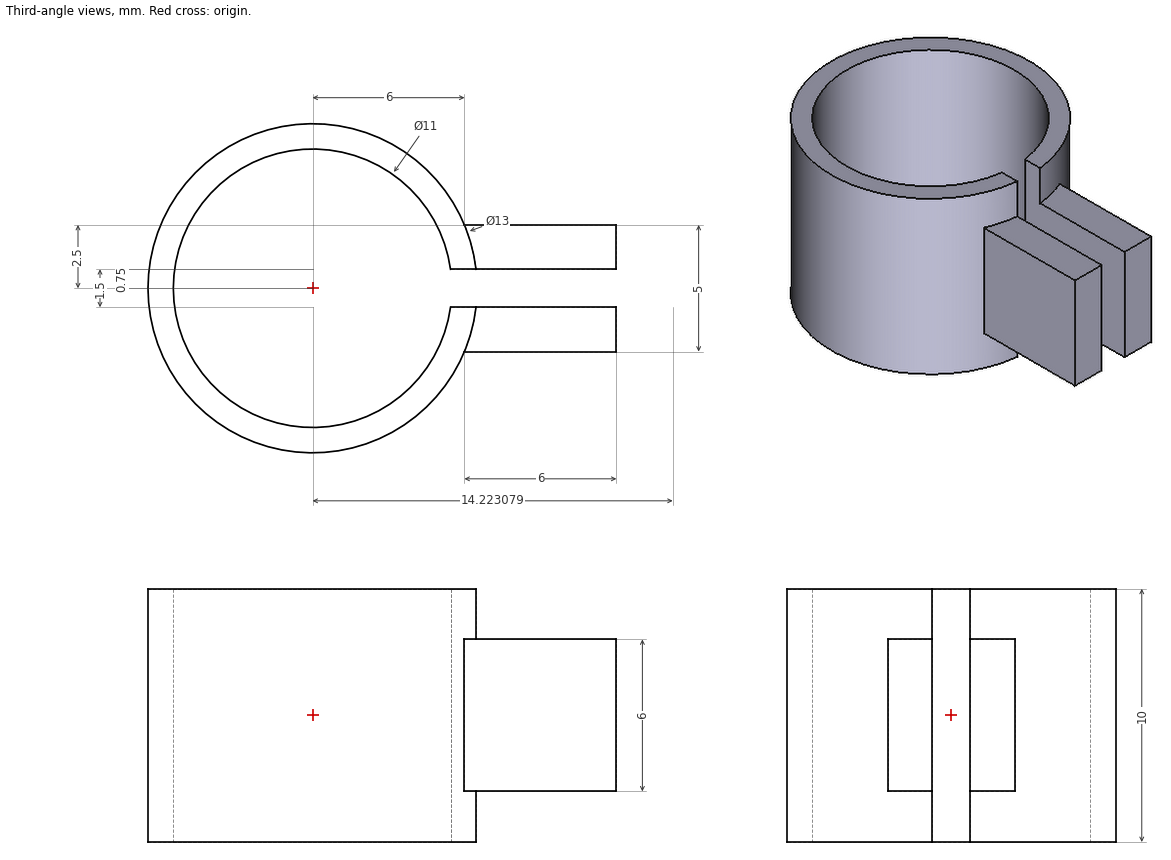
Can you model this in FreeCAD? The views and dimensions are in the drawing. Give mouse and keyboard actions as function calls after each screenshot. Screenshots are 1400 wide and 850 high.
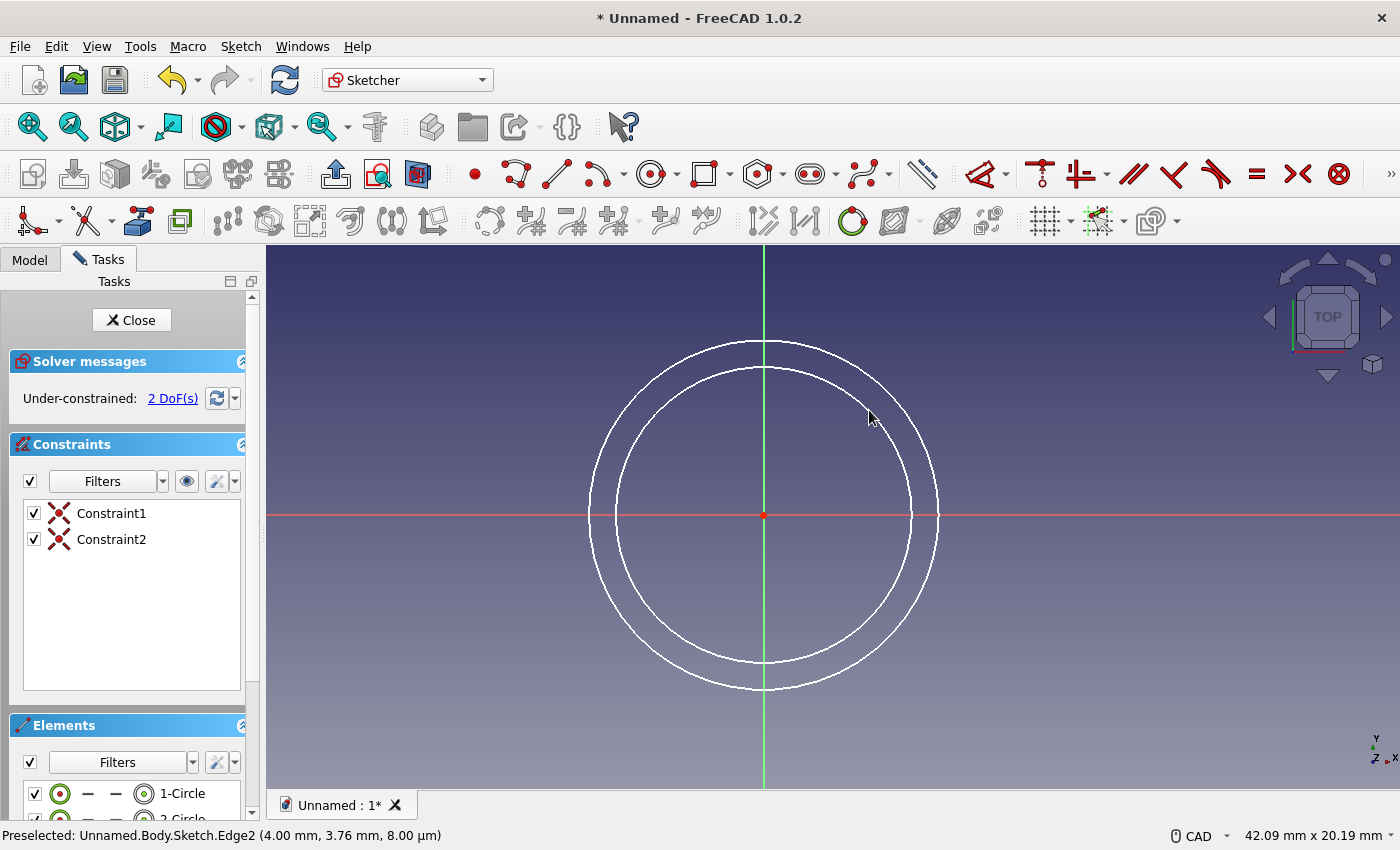
key(d)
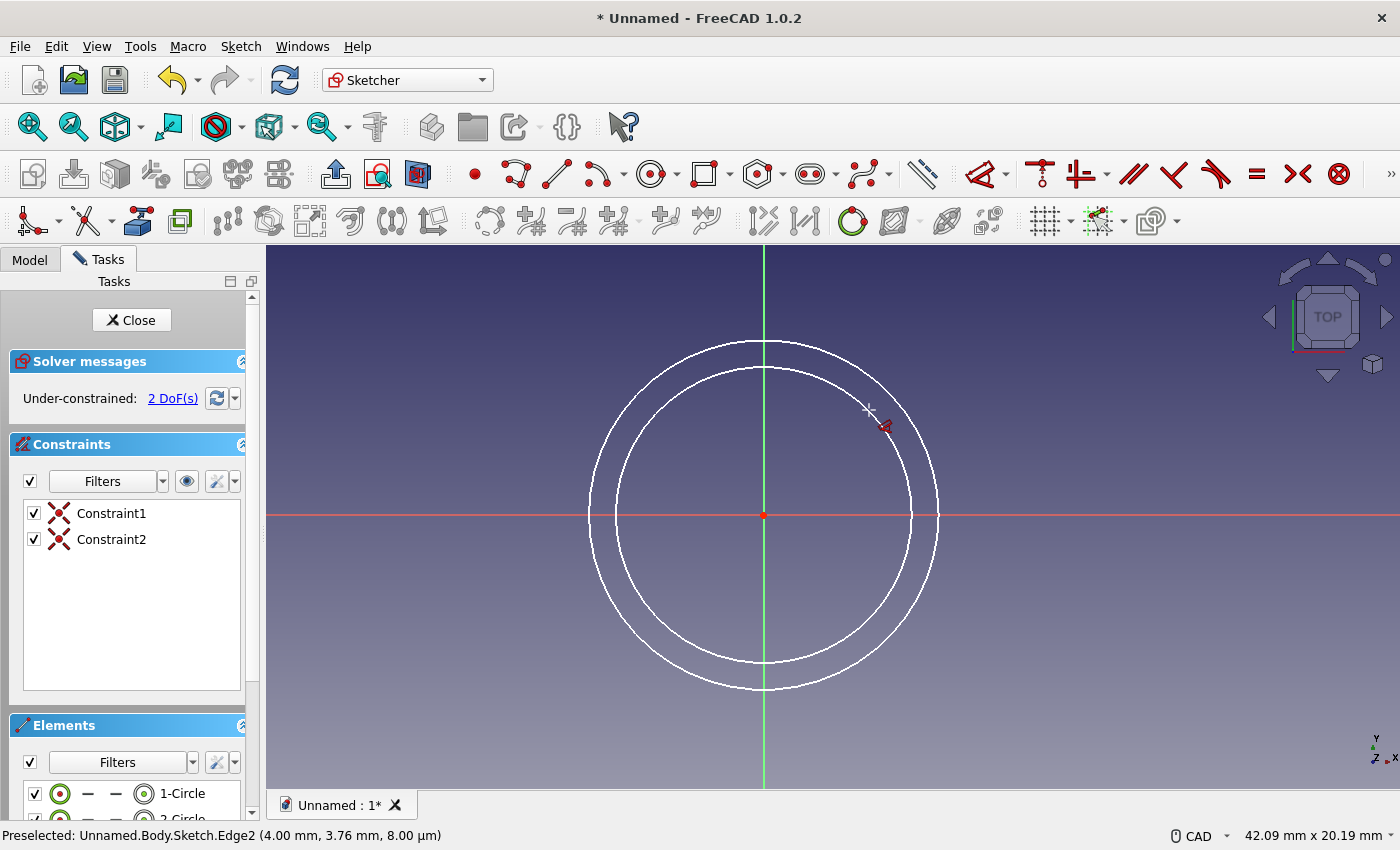
click(887, 391)
click(910, 368)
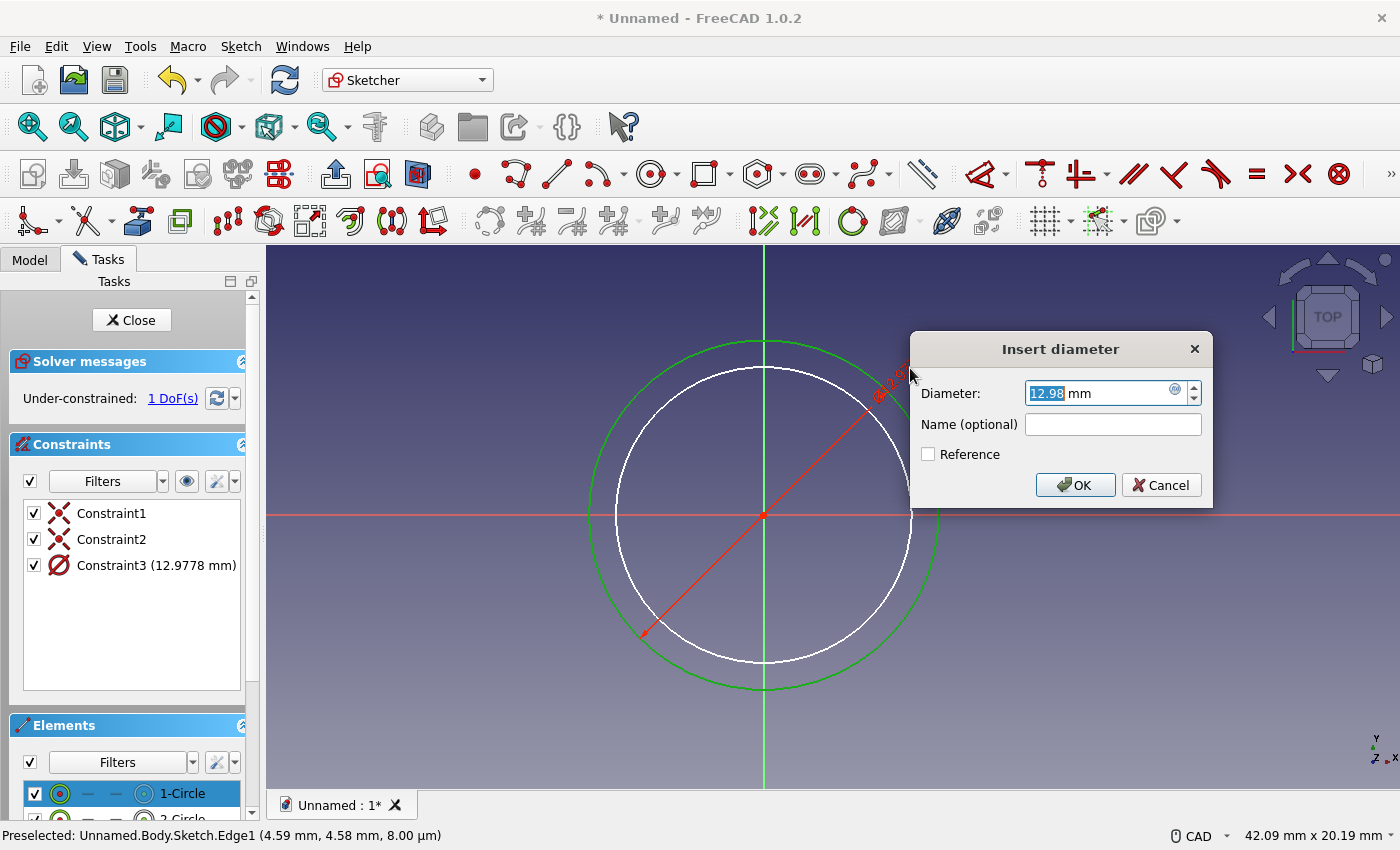
text(13)
key(Return)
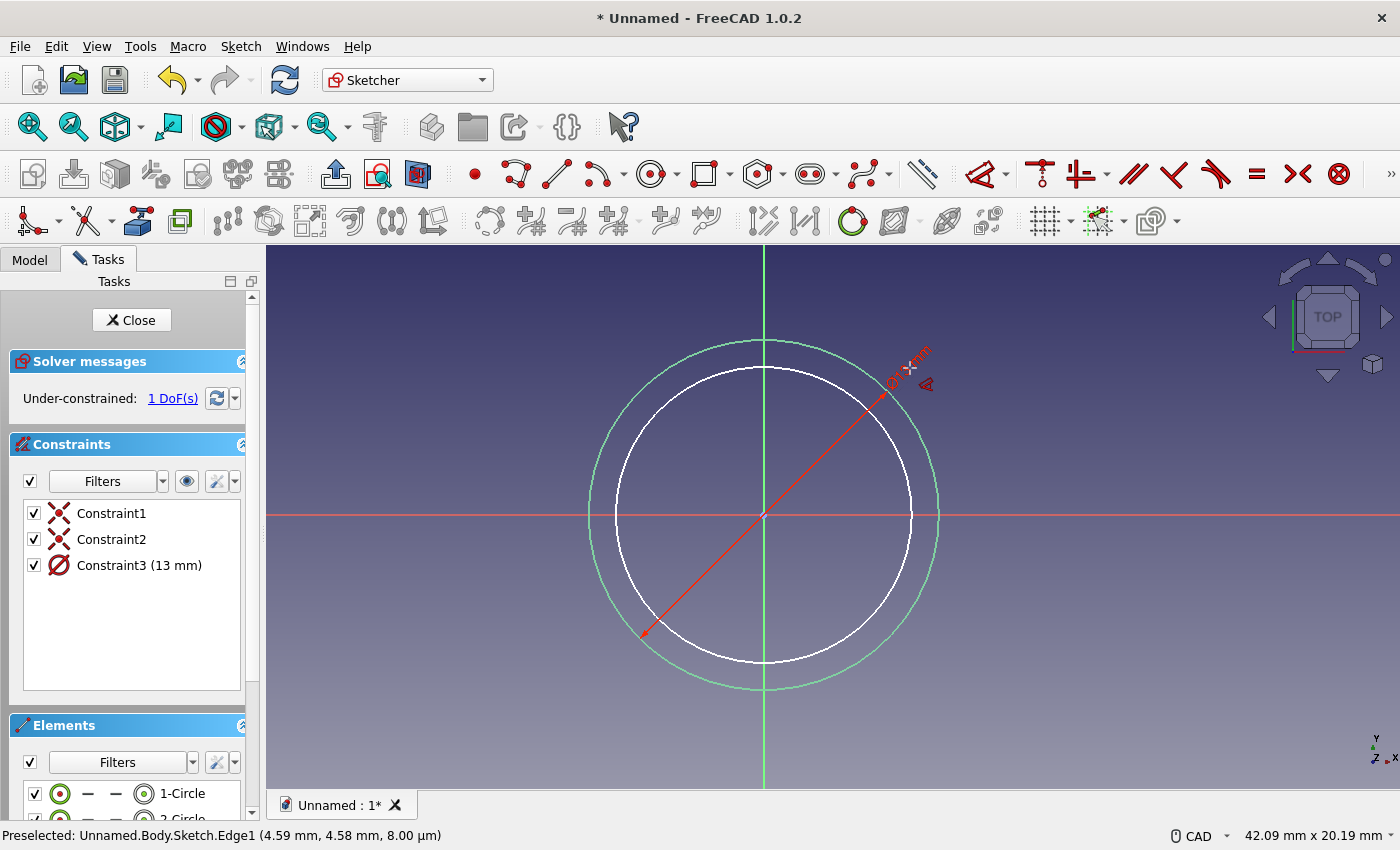
click(868, 410)
click(958, 457)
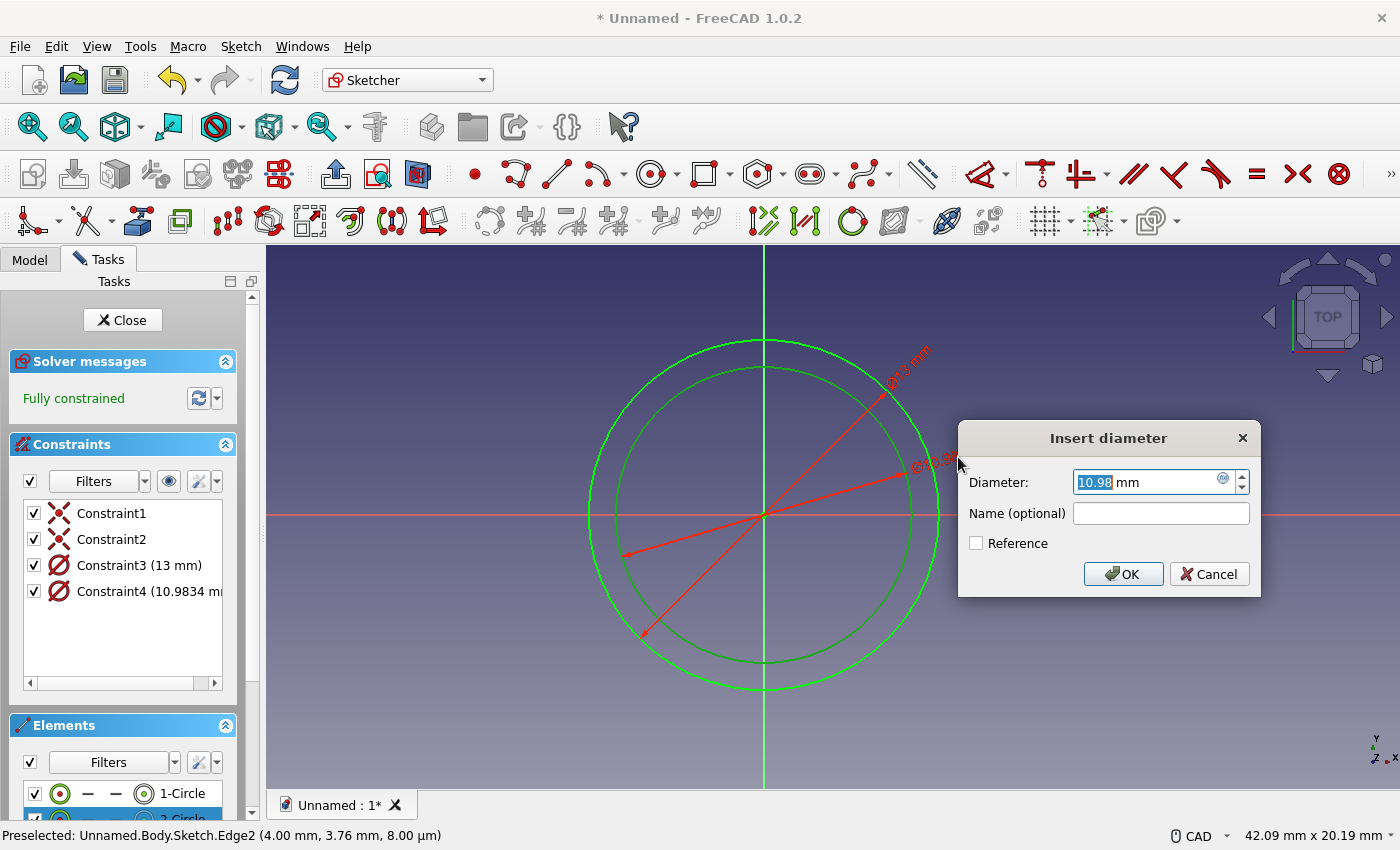
text(11)
key(Return)
key(Escape)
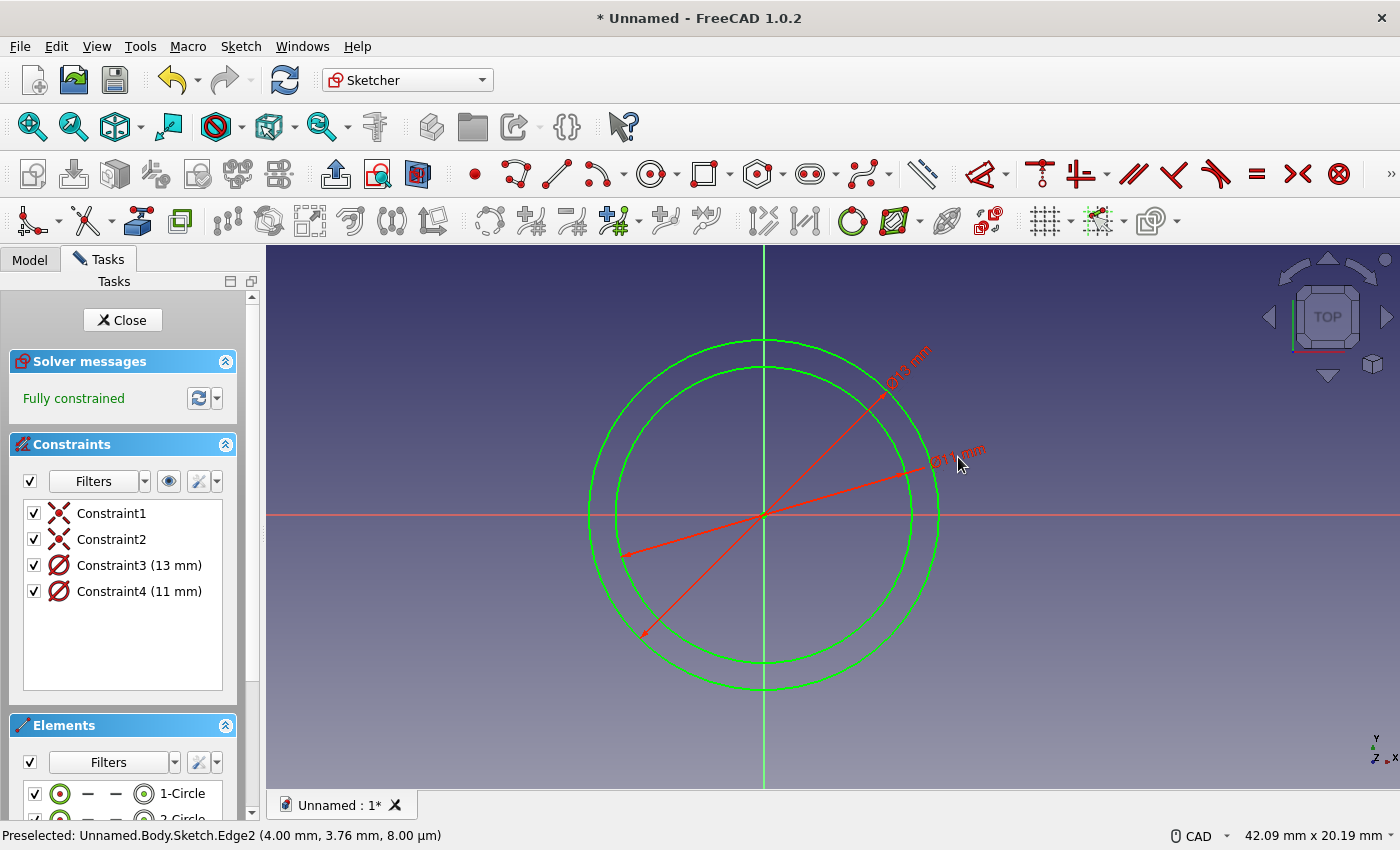
click(123, 320)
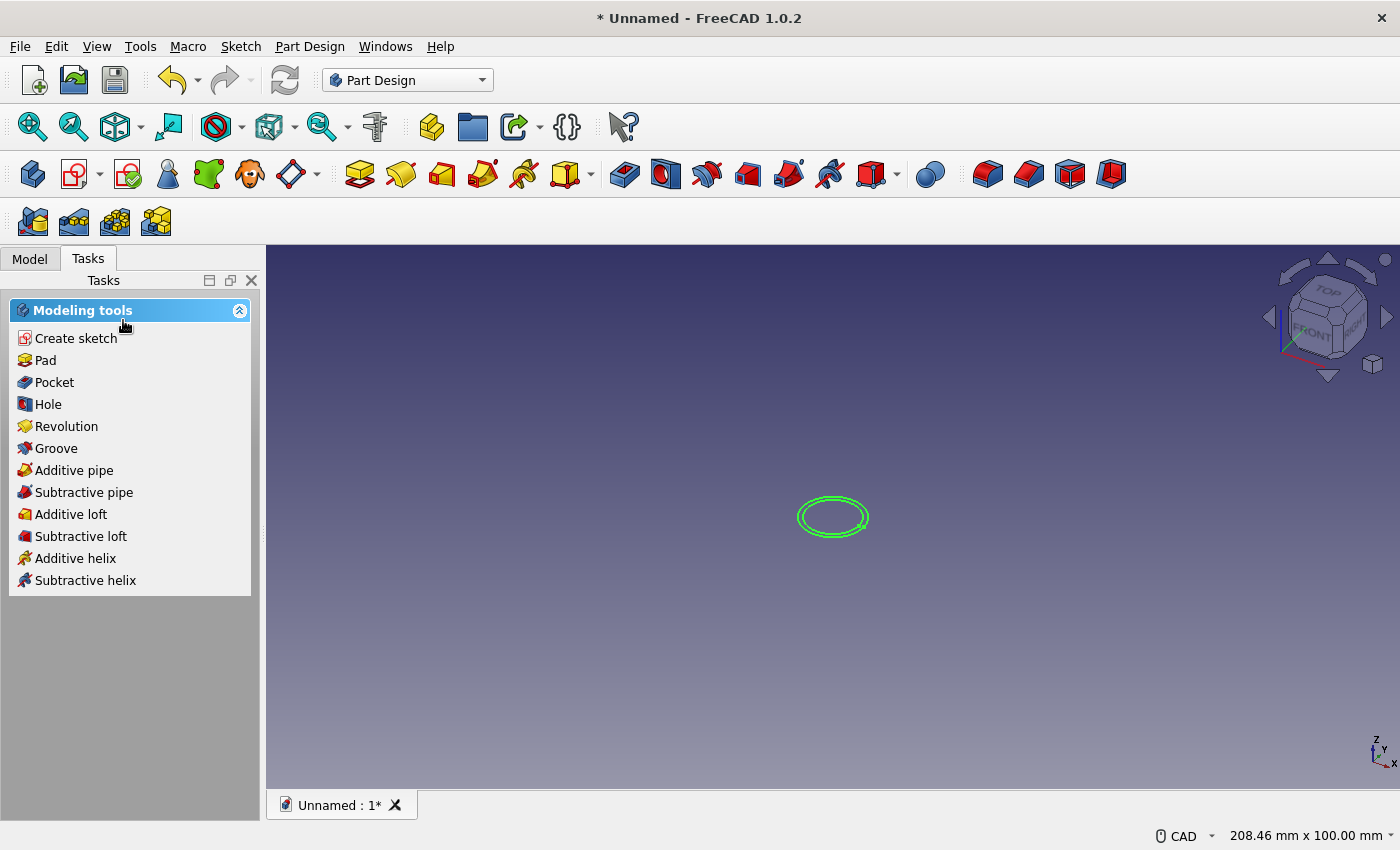
click(360, 174)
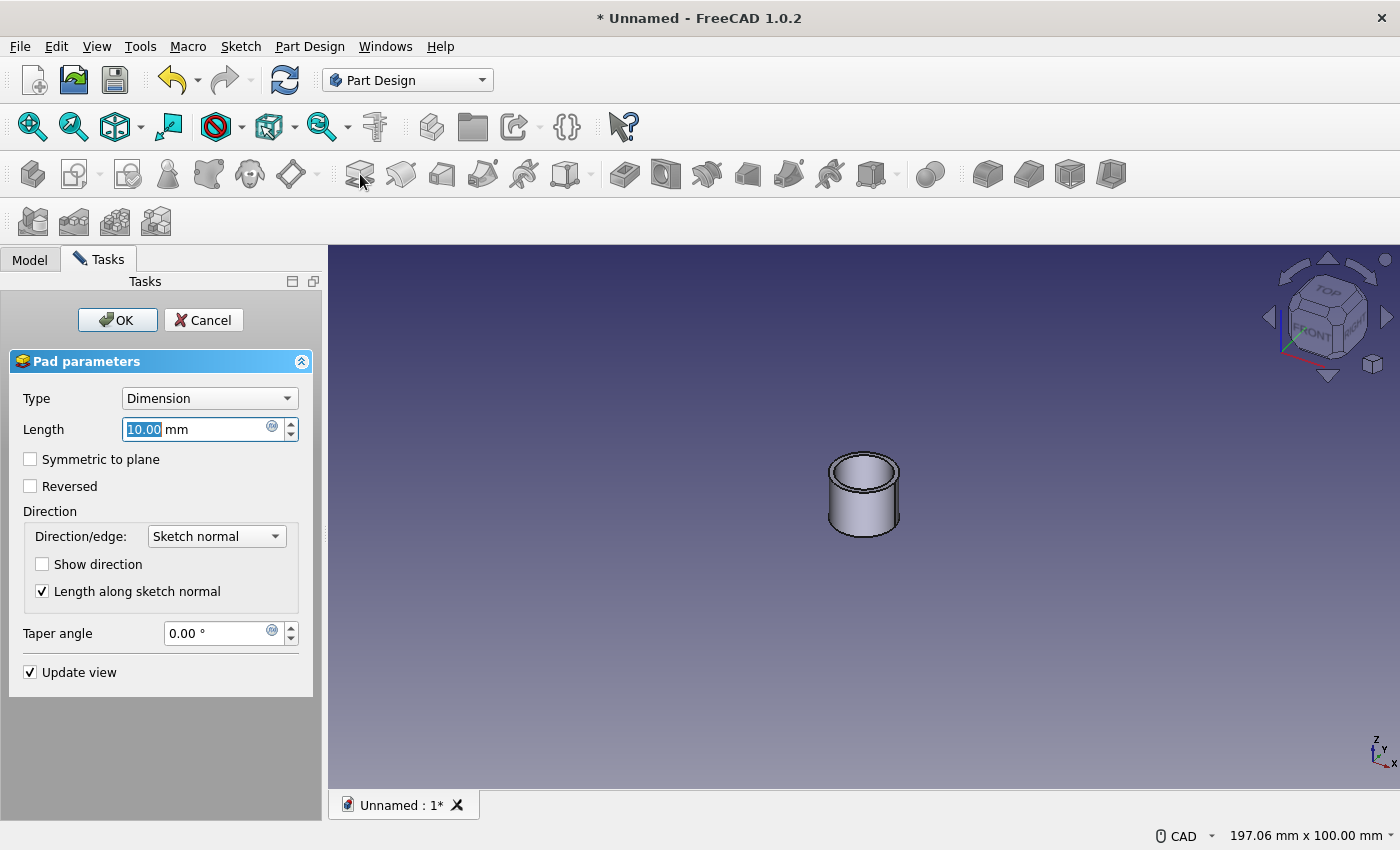
text(10)
key(Tab)